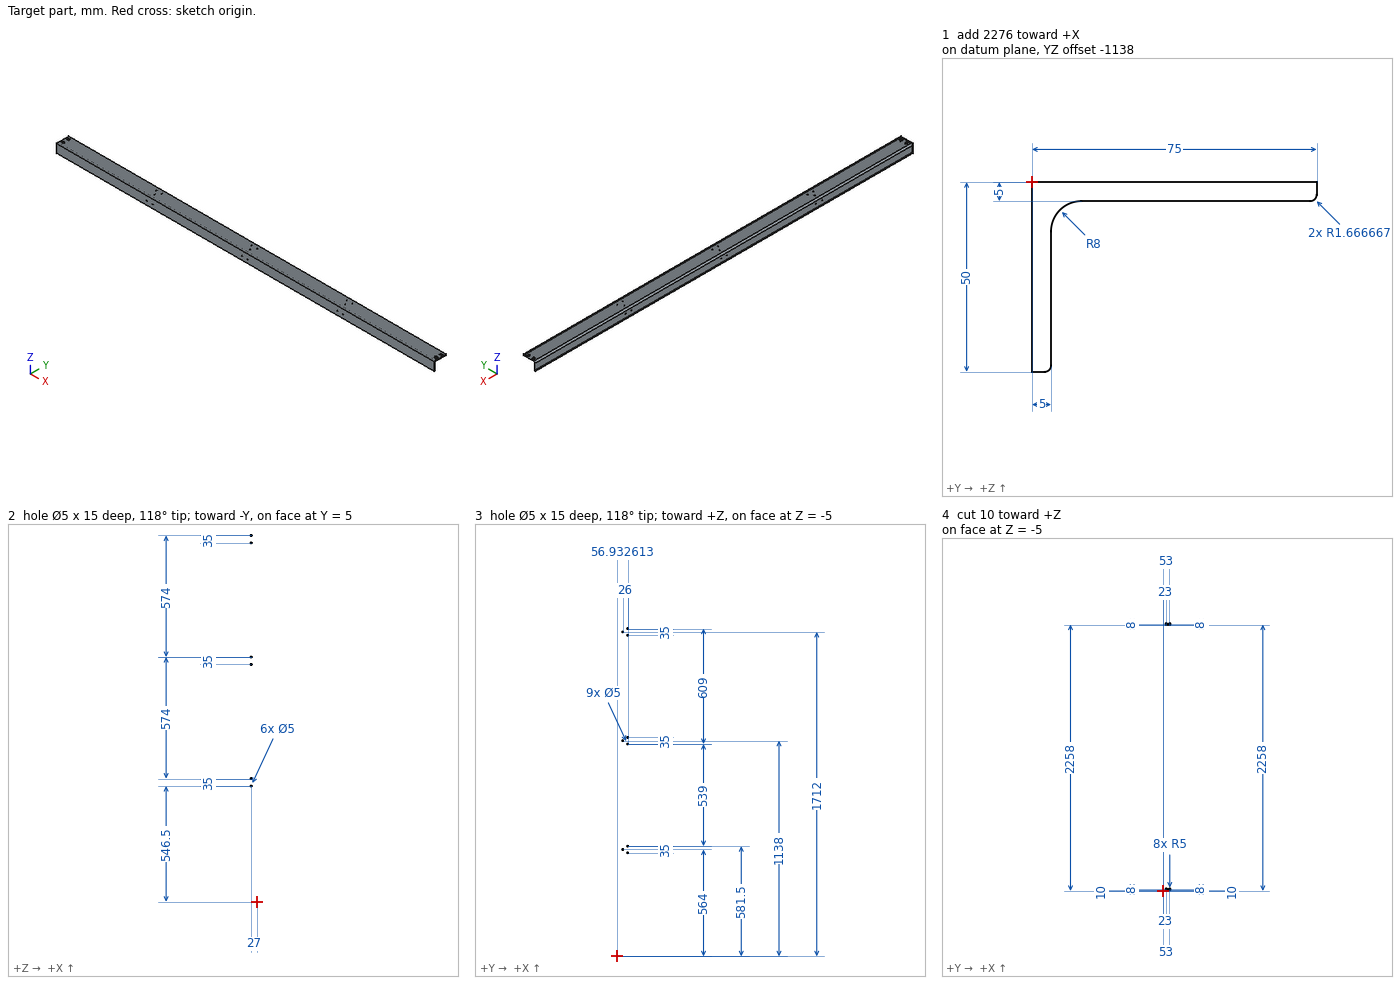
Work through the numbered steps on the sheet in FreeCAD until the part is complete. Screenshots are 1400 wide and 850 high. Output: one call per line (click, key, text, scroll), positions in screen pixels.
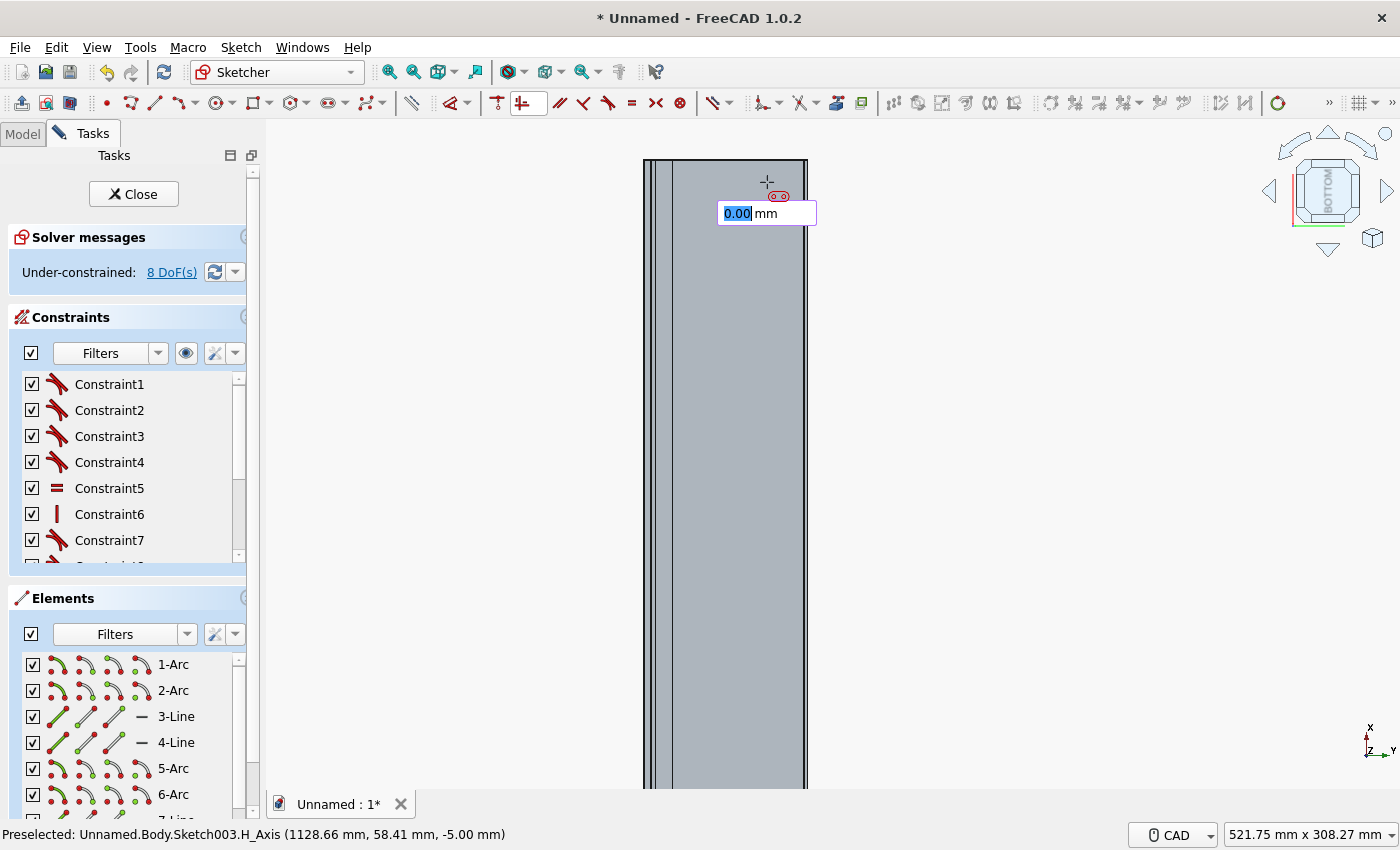
scroll(781, 190, up, 2)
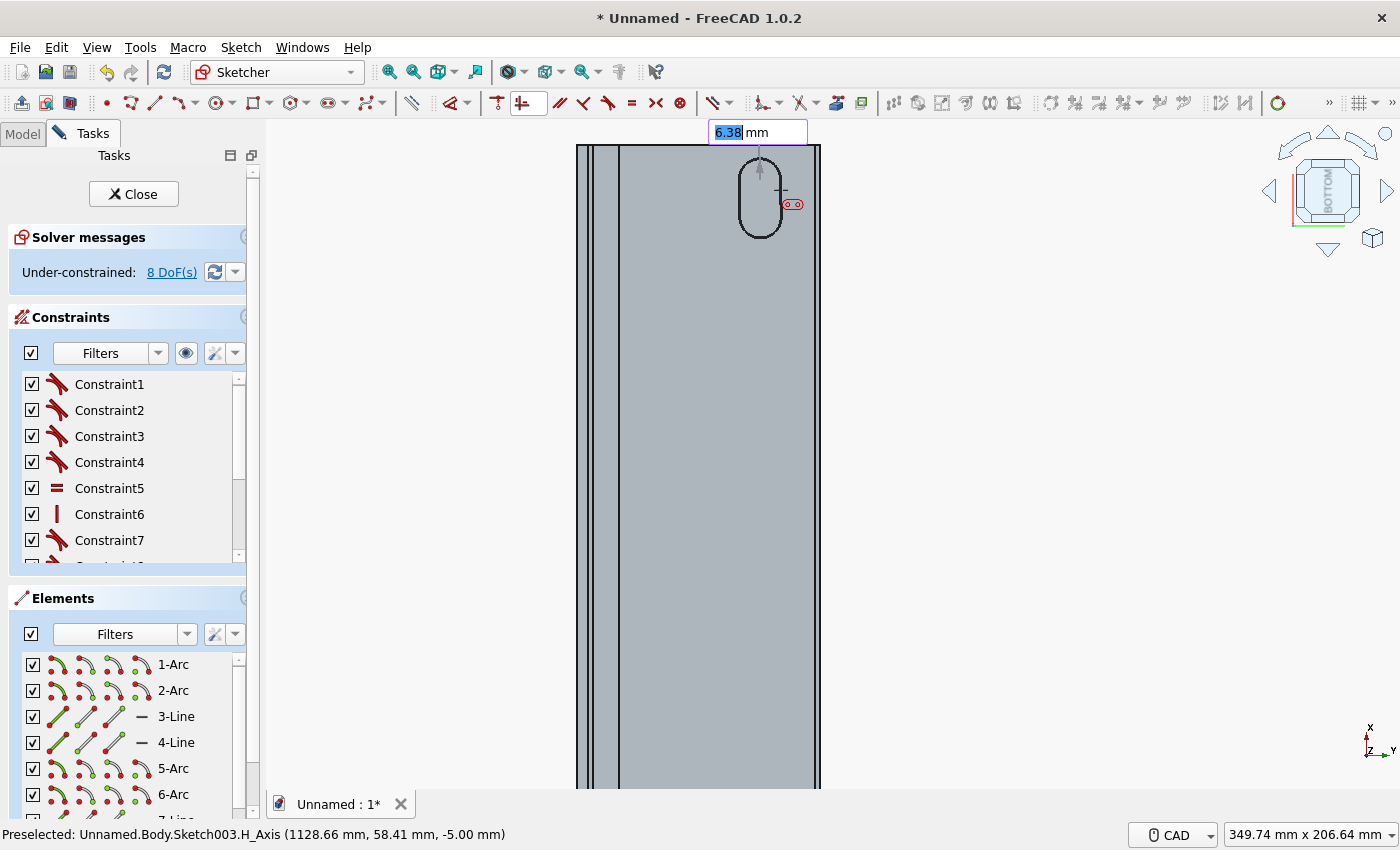
click(781, 191)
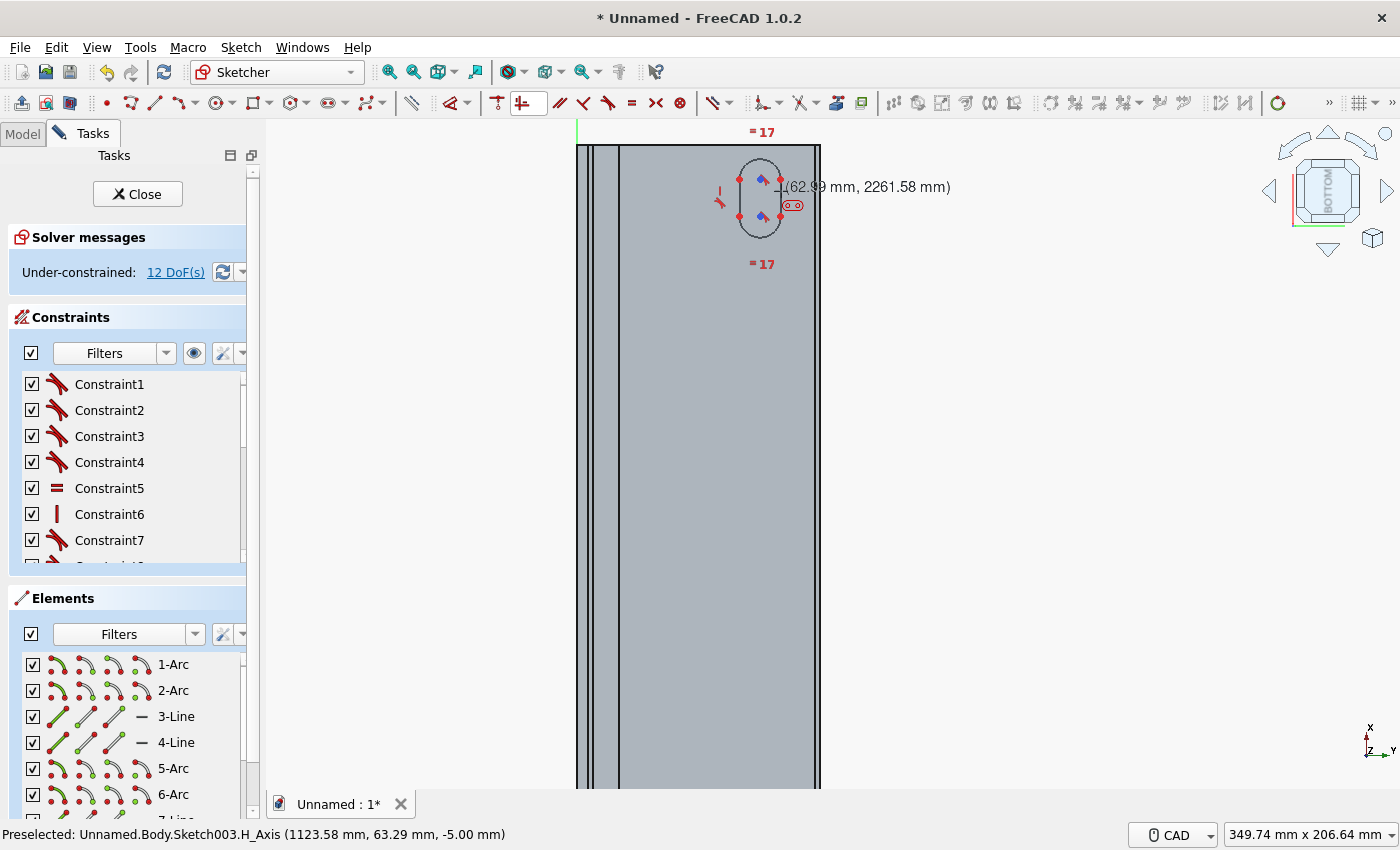
scroll(668, 204, up, 2)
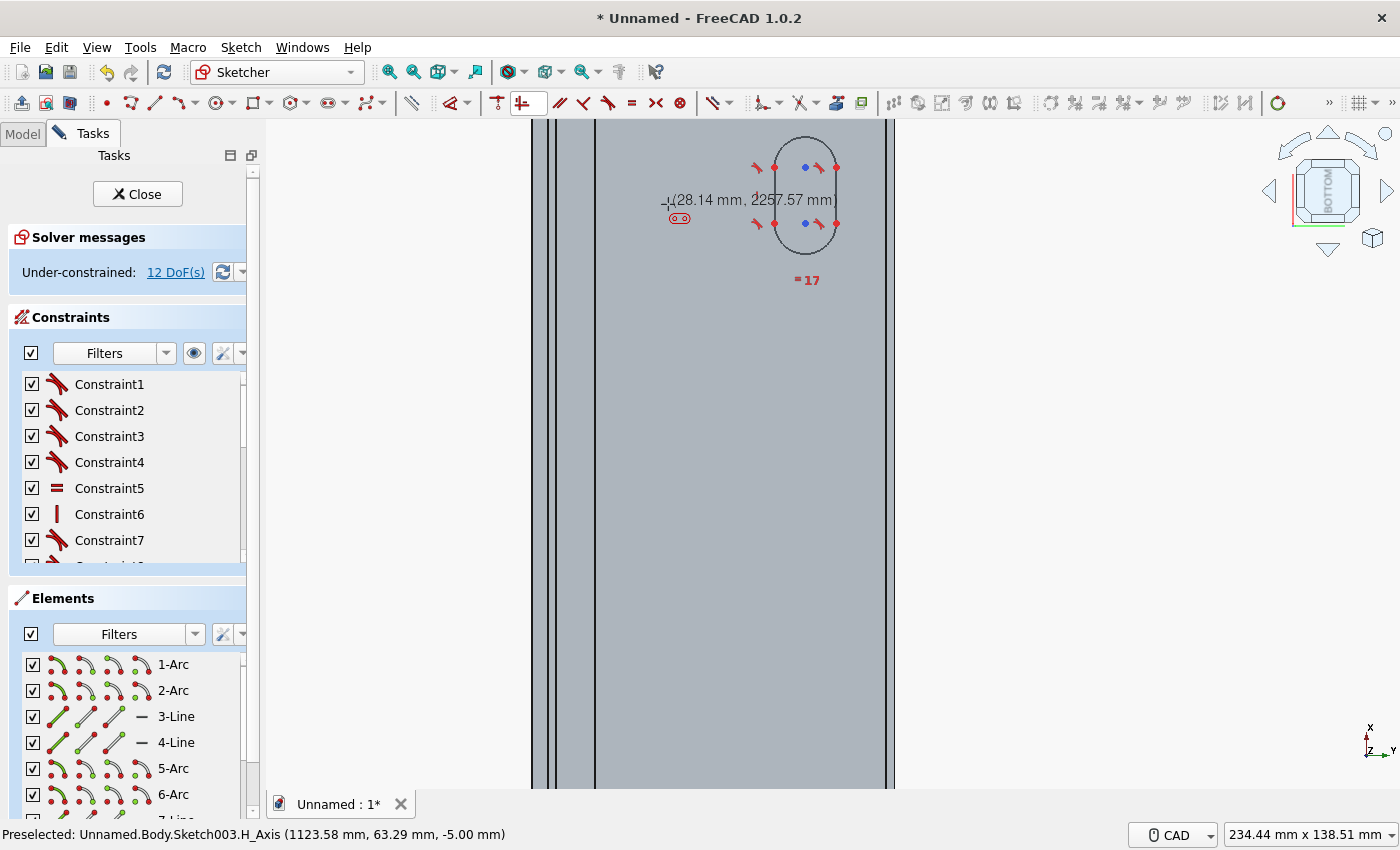
scroll(769, 183, down, 15)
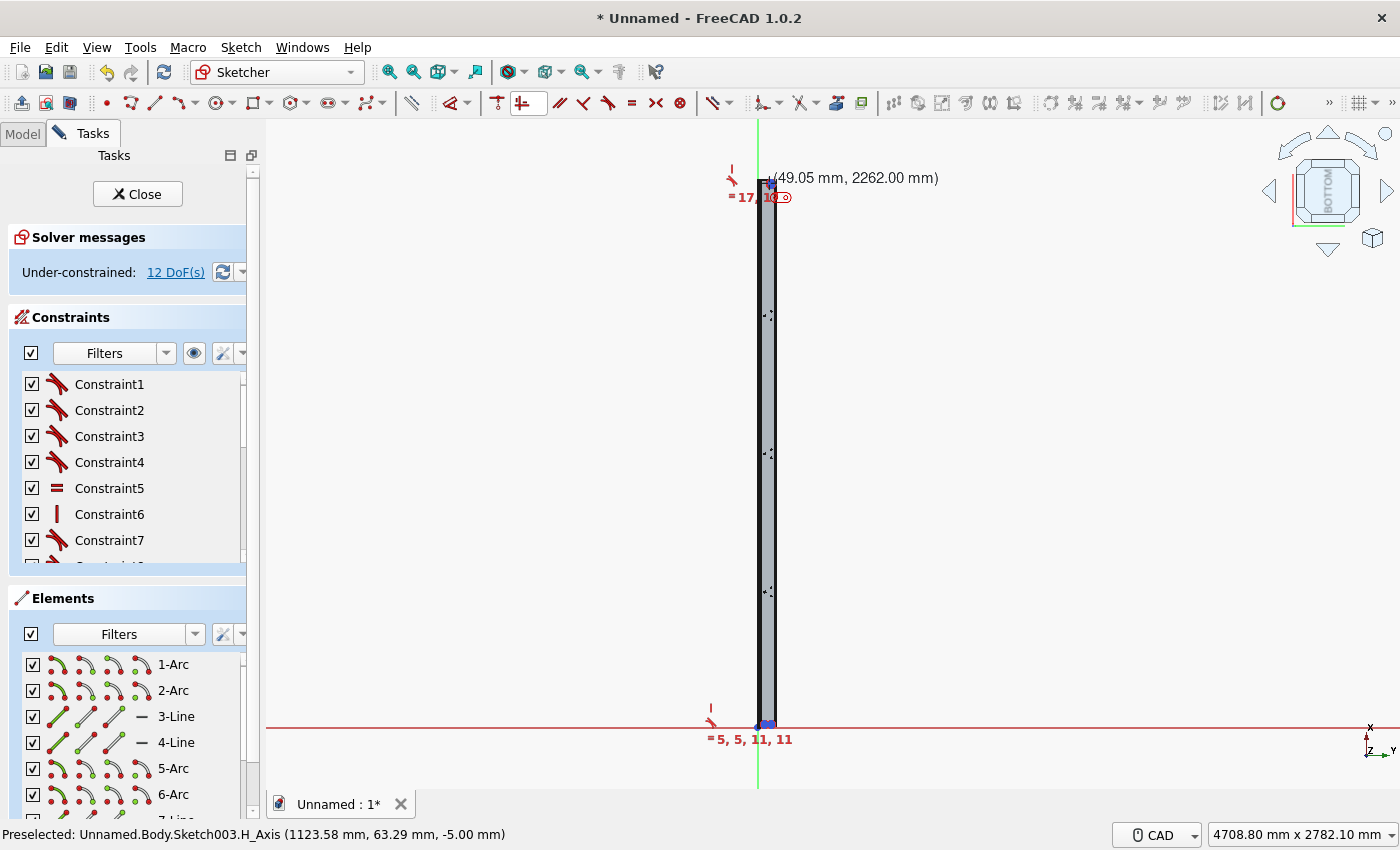
scroll(764, 184, up, 5)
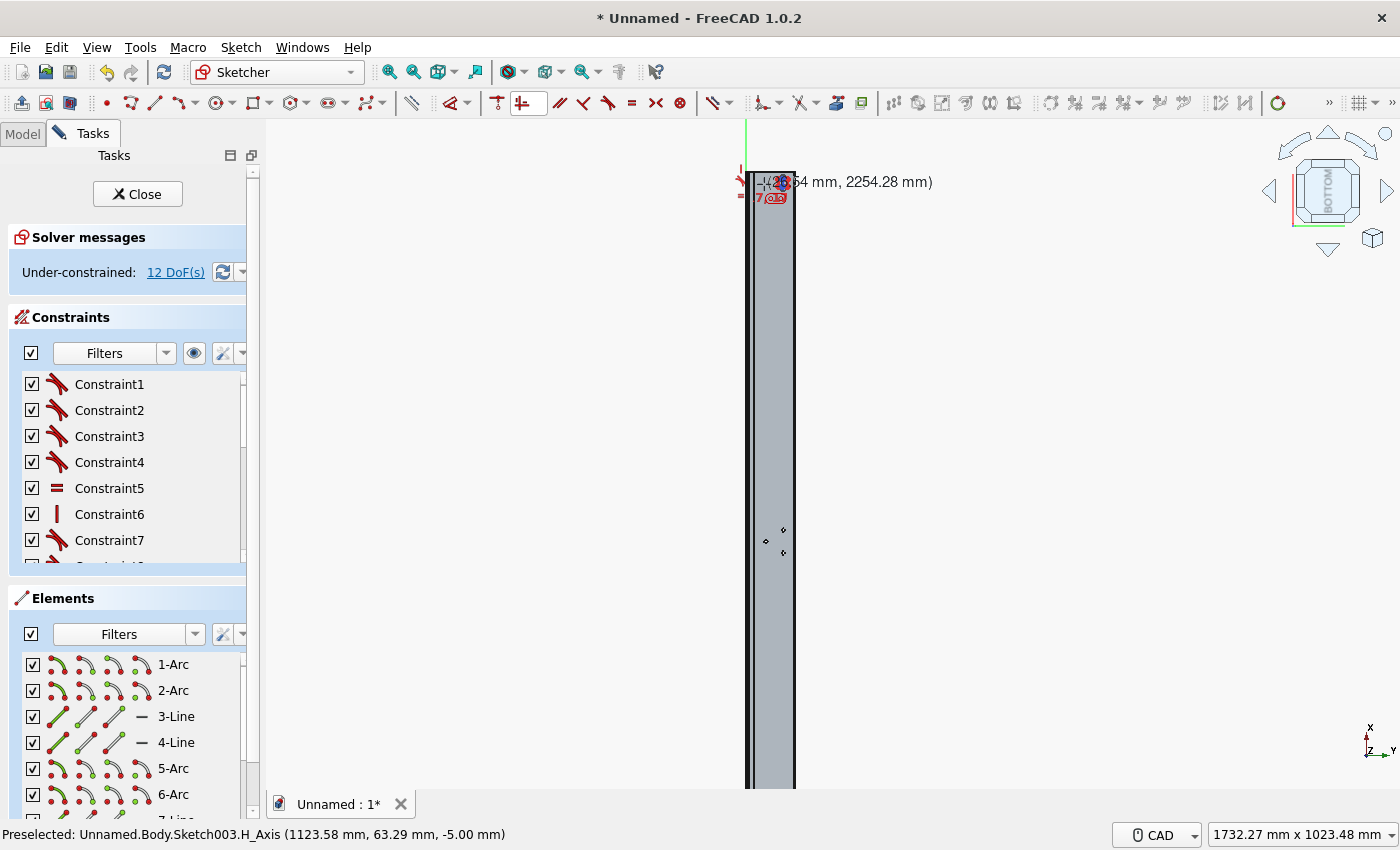
click(764, 184)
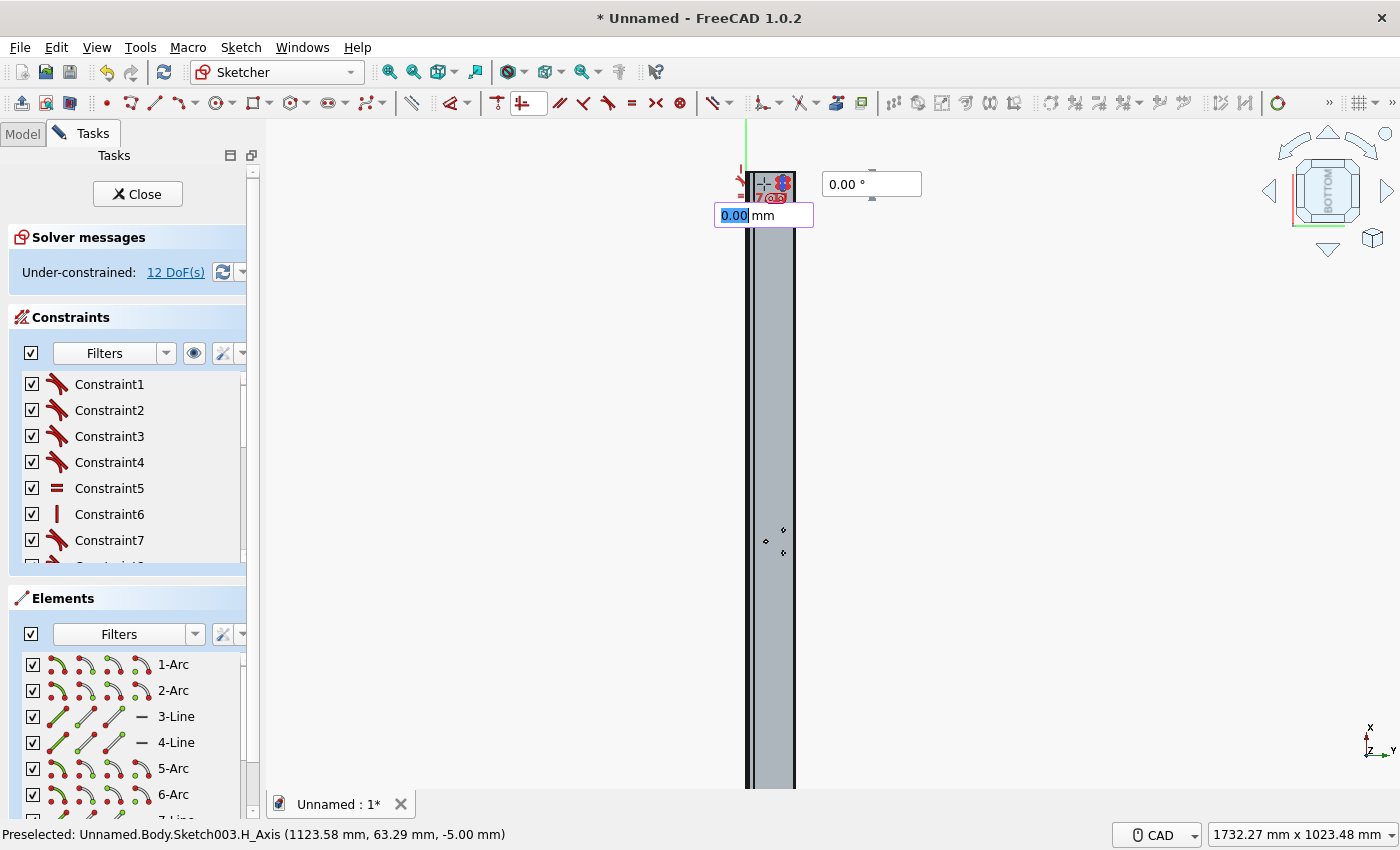
scroll(764, 179, up, 6)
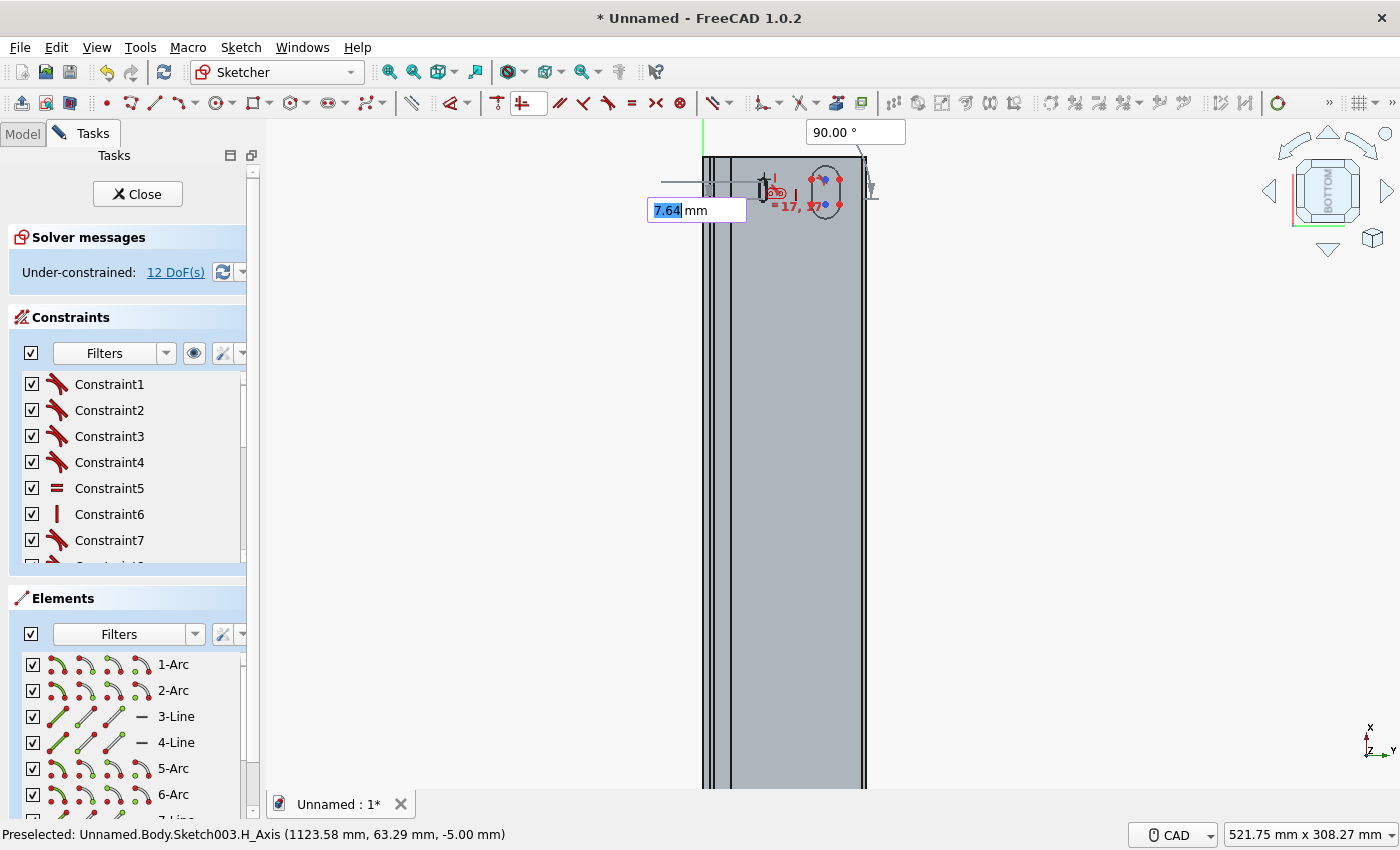
click(763, 178)